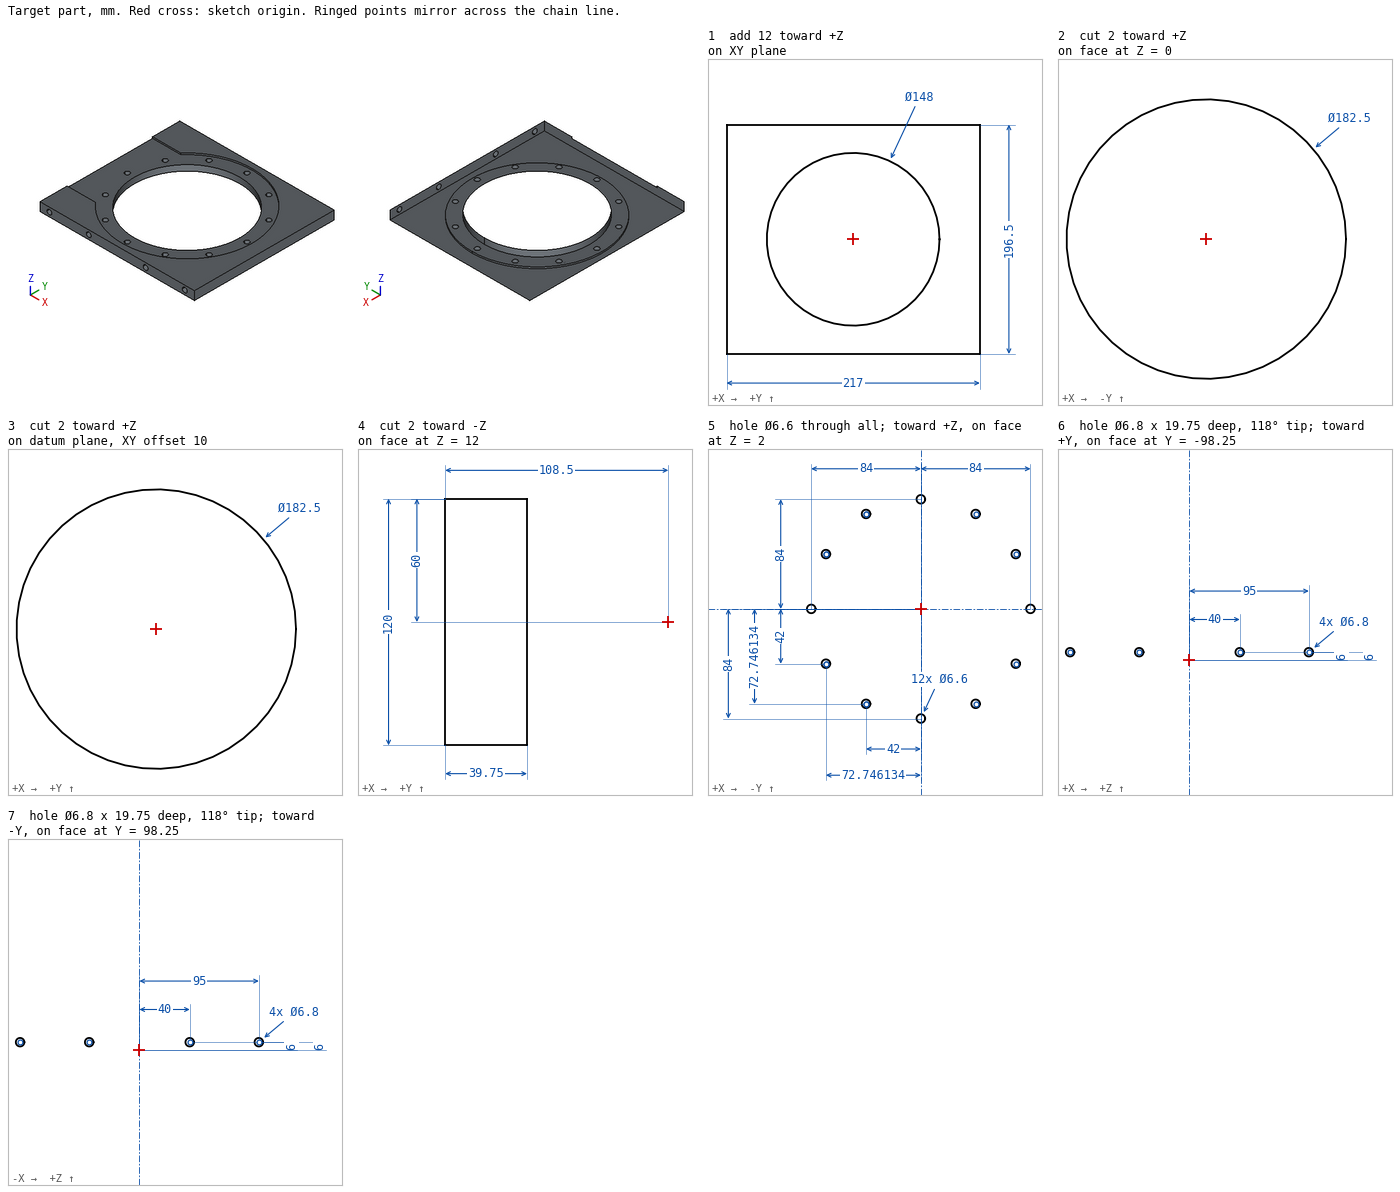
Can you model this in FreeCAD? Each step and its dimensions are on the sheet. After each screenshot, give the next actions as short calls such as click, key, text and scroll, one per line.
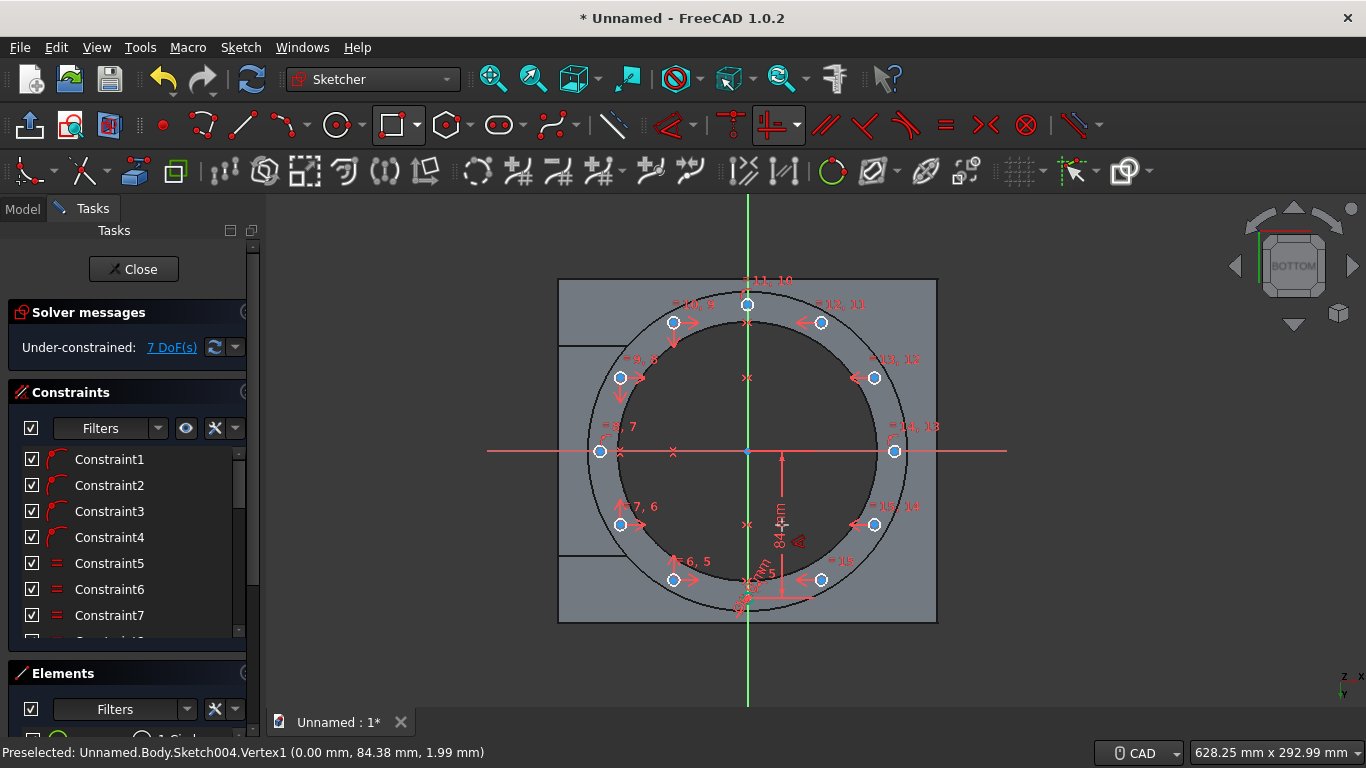
click(674, 580)
click(711, 614)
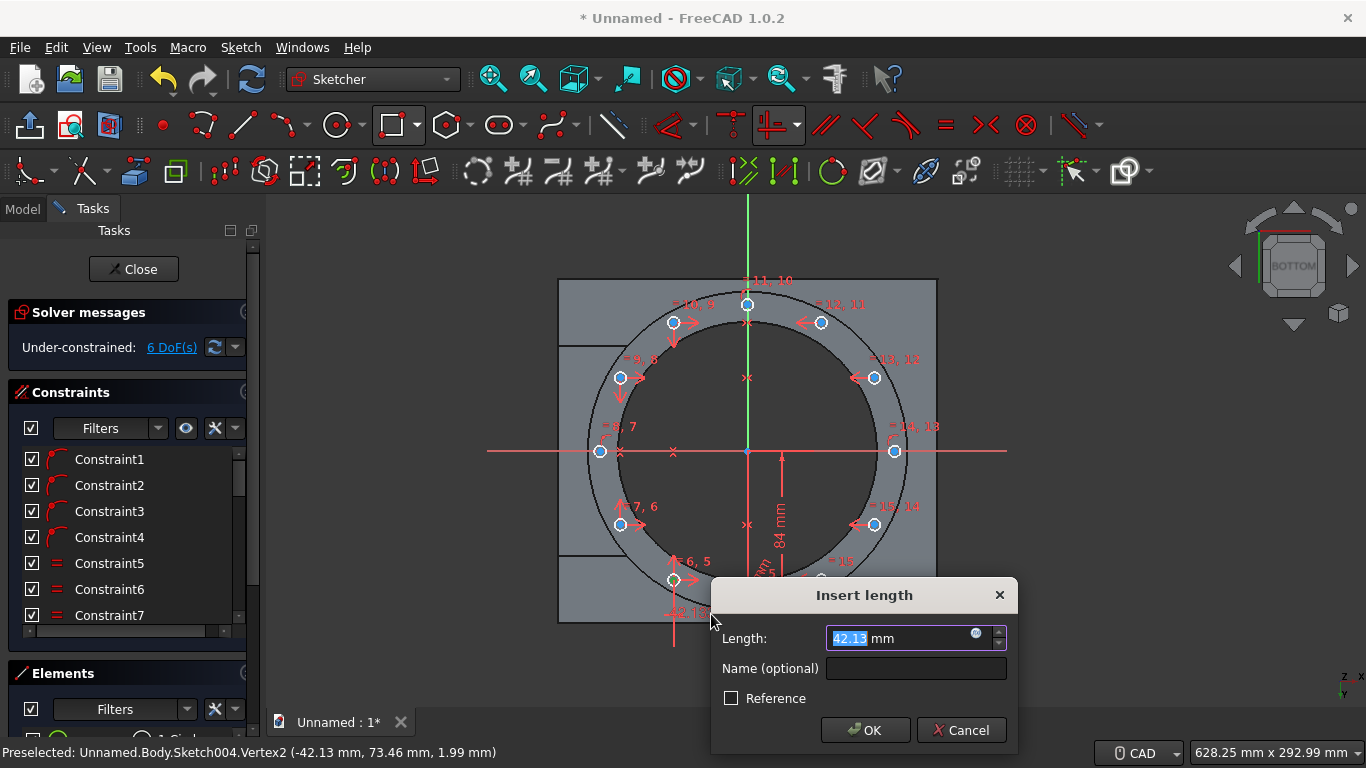
text(42)
key(Return)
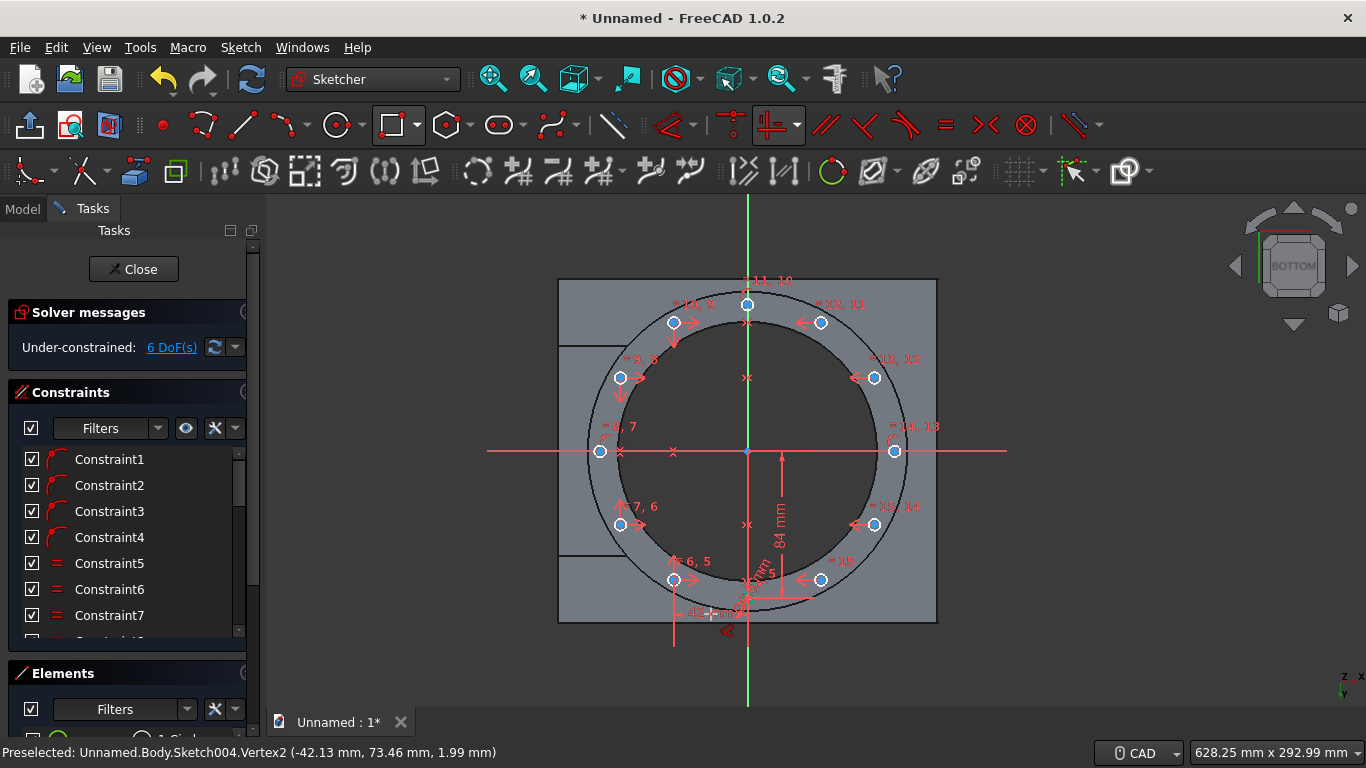
click(620, 525)
click(586, 488)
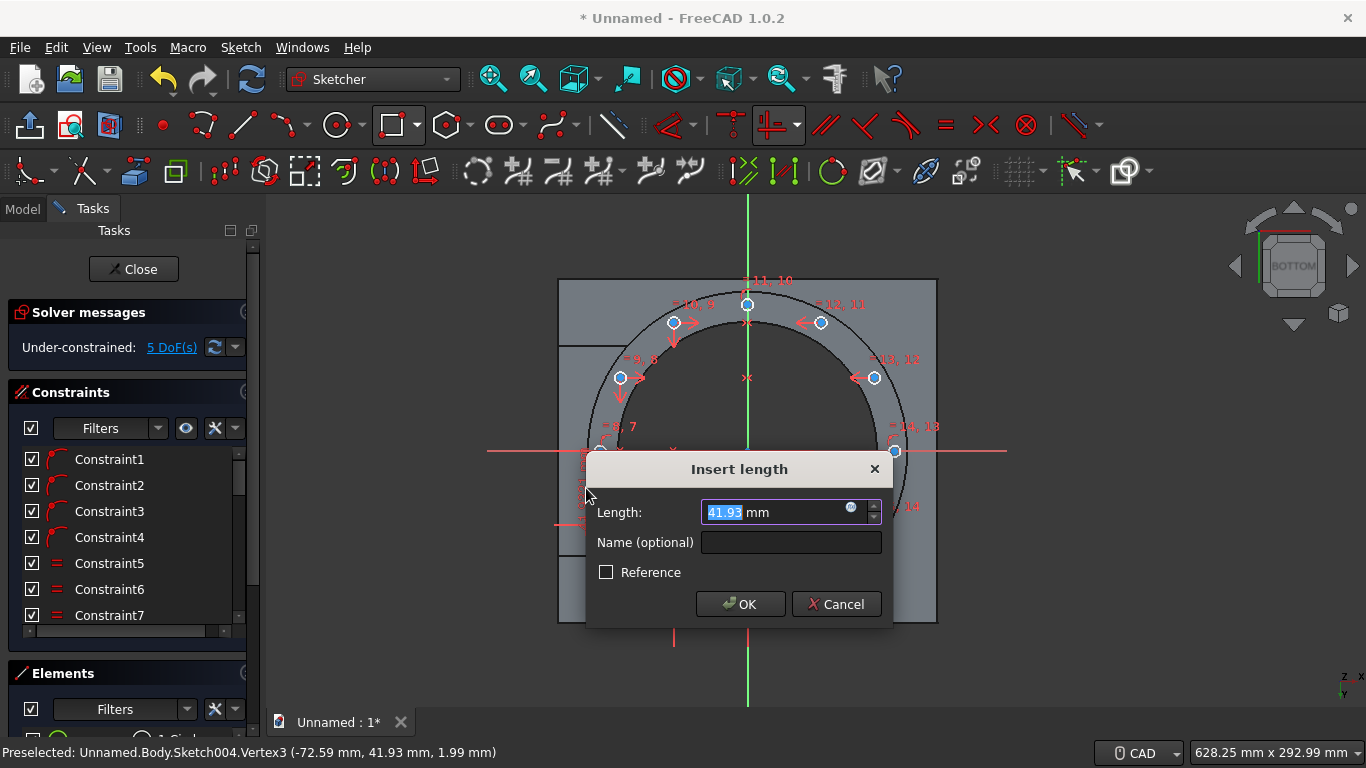
text(42)
key(Return)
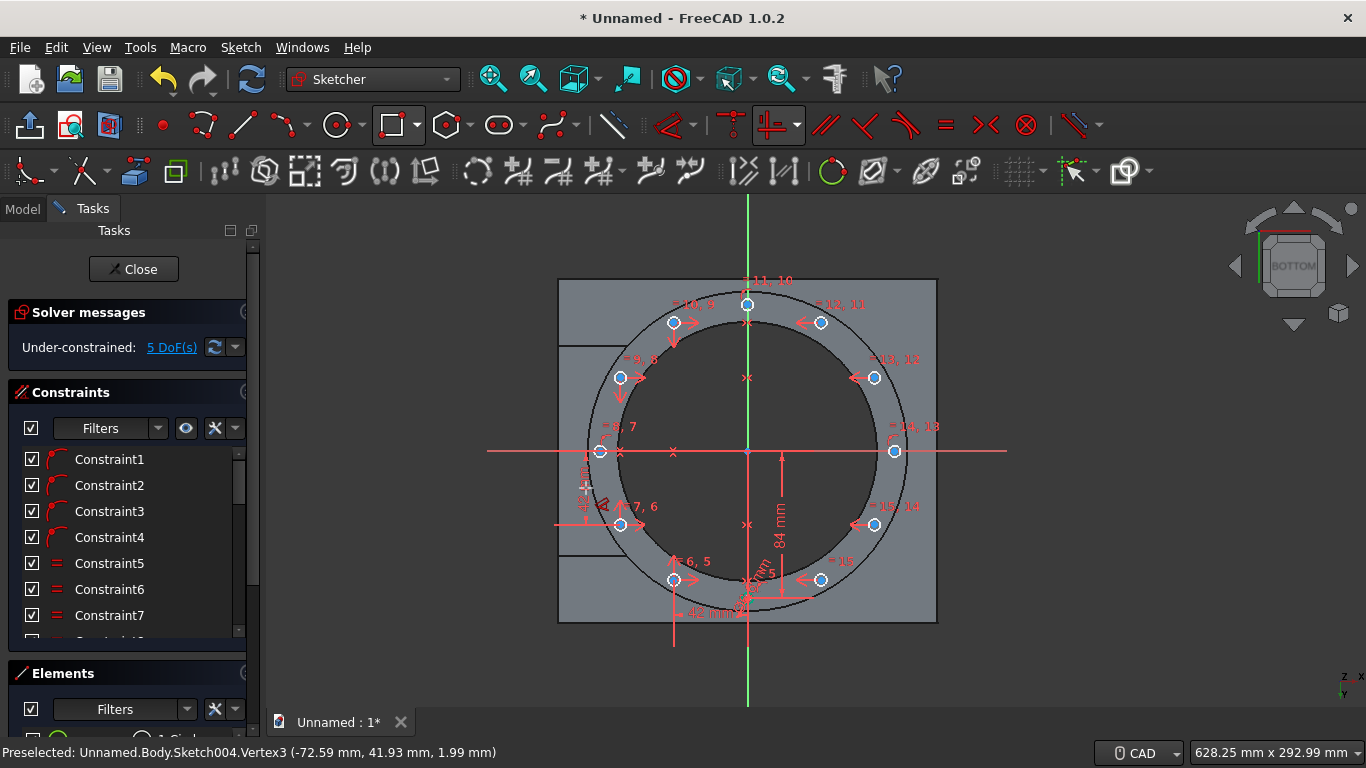
click(600, 451)
click(674, 485)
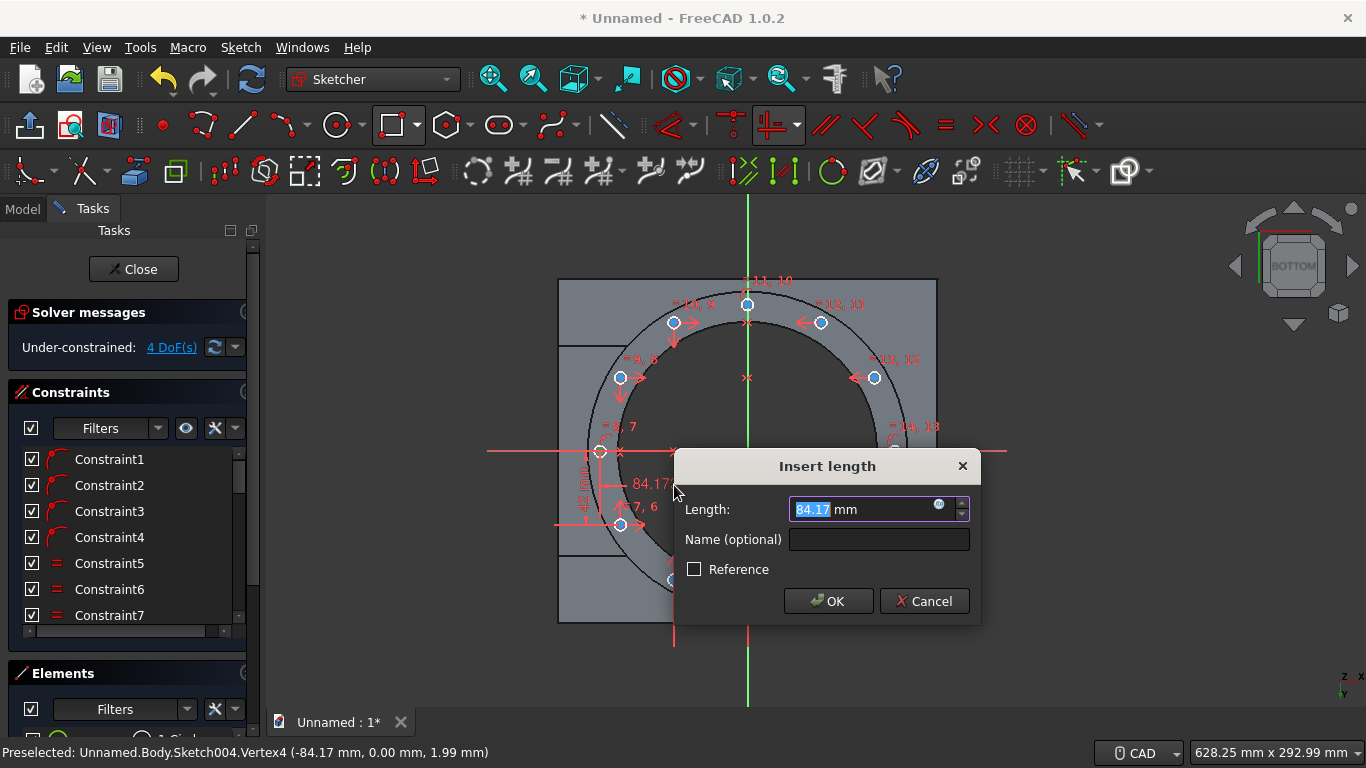
text(84)
key(Return)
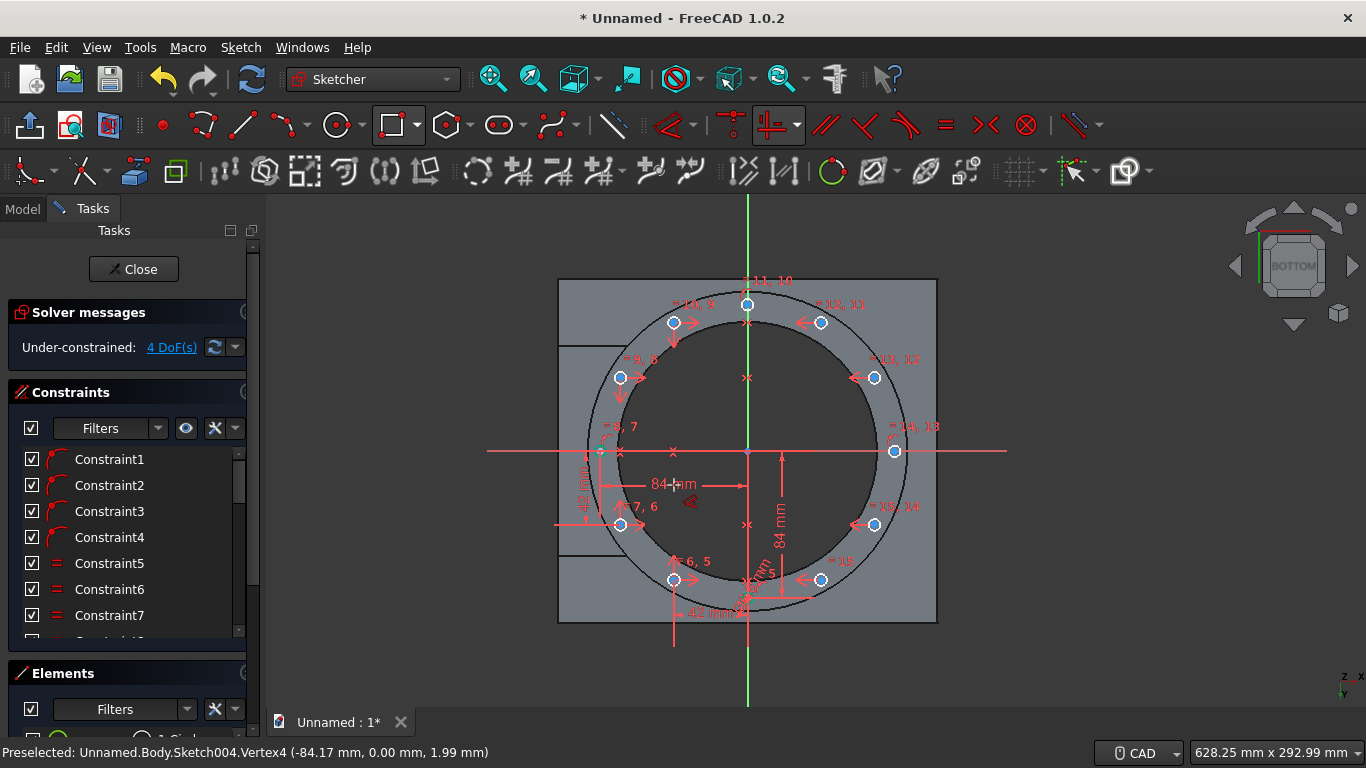
click(748, 305)
click(782, 378)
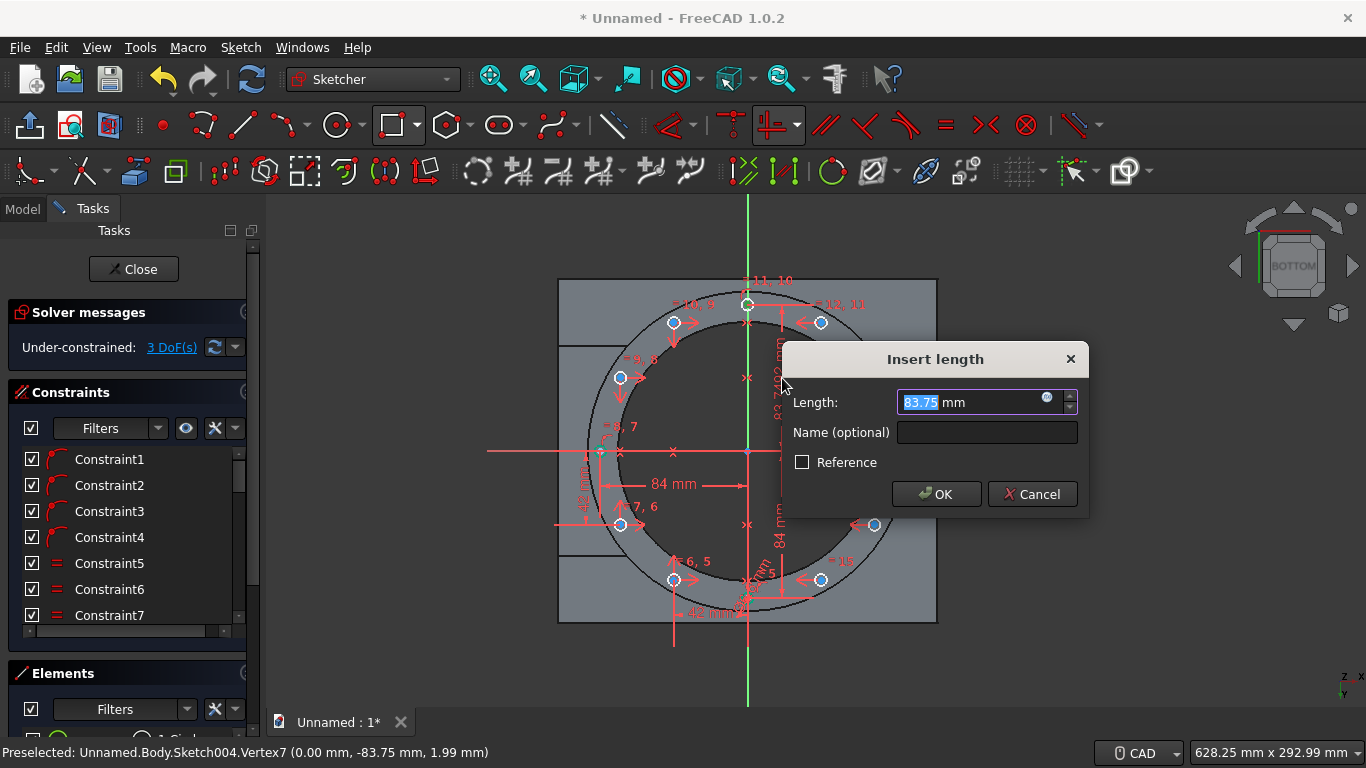
text(84)
key(Return)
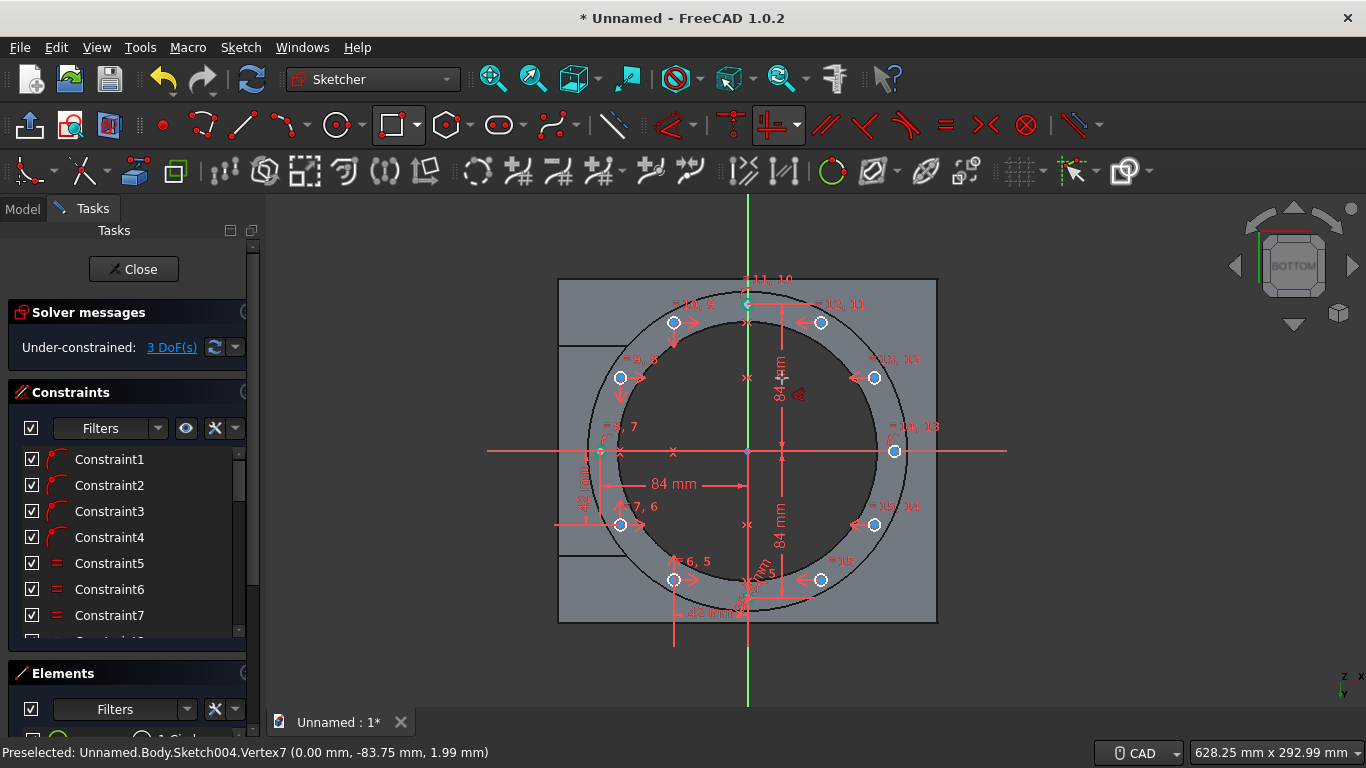
click(895, 451)
click(821, 485)